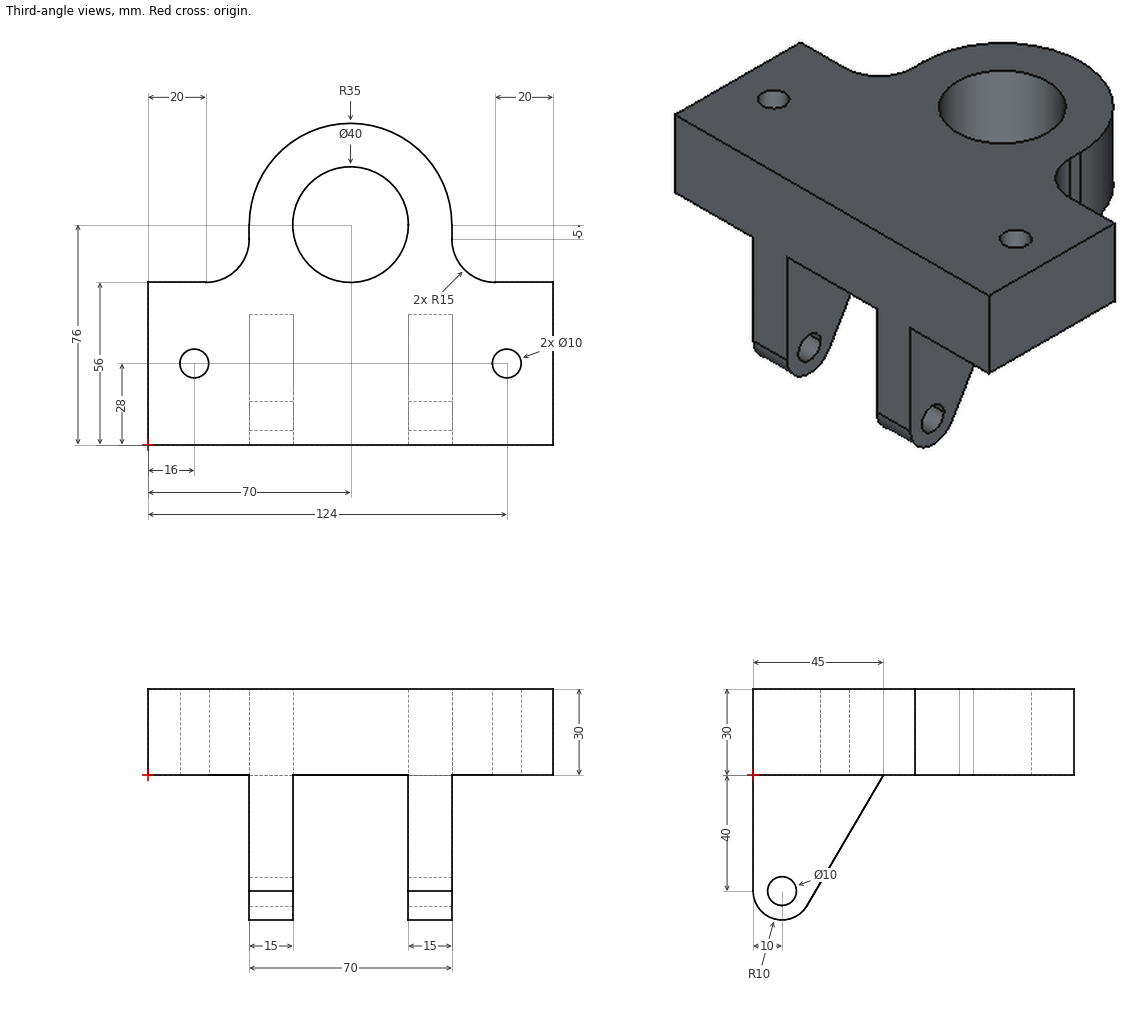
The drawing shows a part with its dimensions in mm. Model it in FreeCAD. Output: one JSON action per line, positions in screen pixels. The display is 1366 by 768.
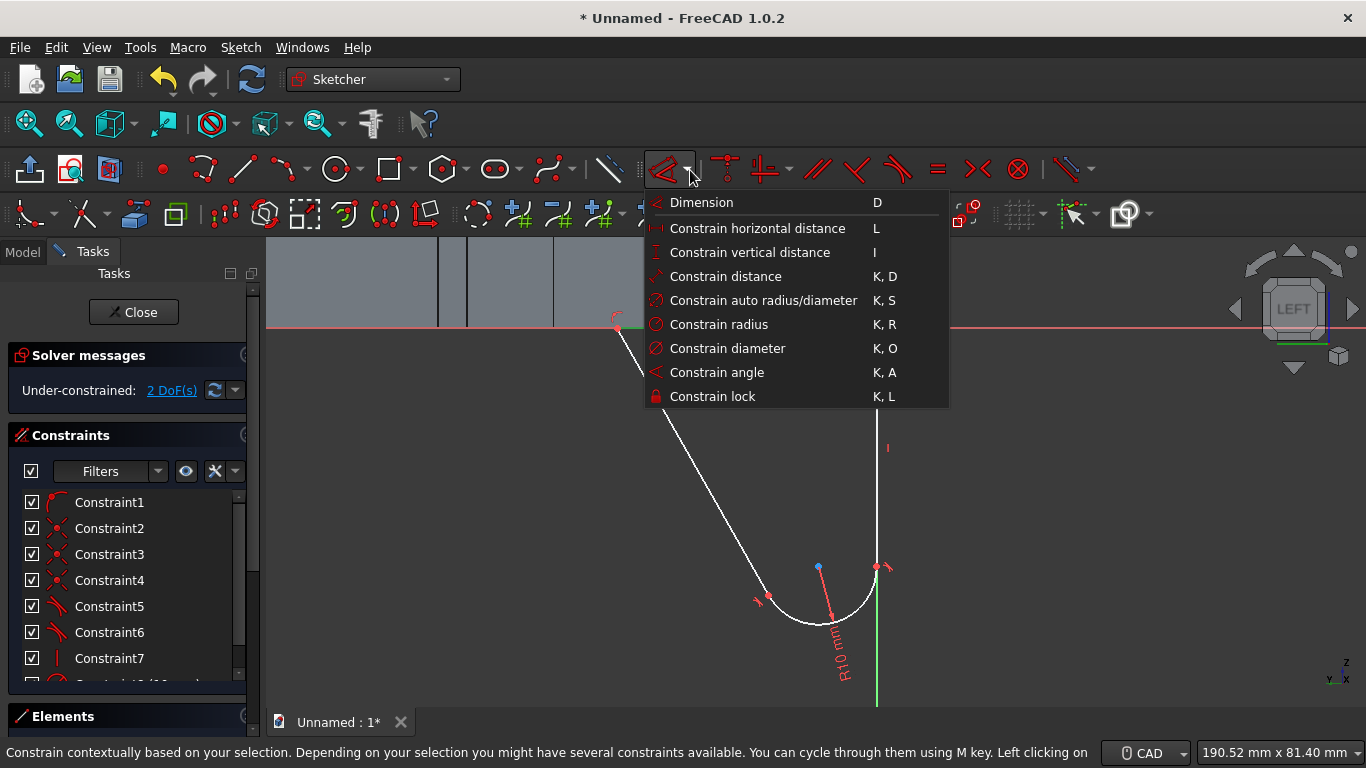
{"action": "left_click", "coordinate": [797, 228]}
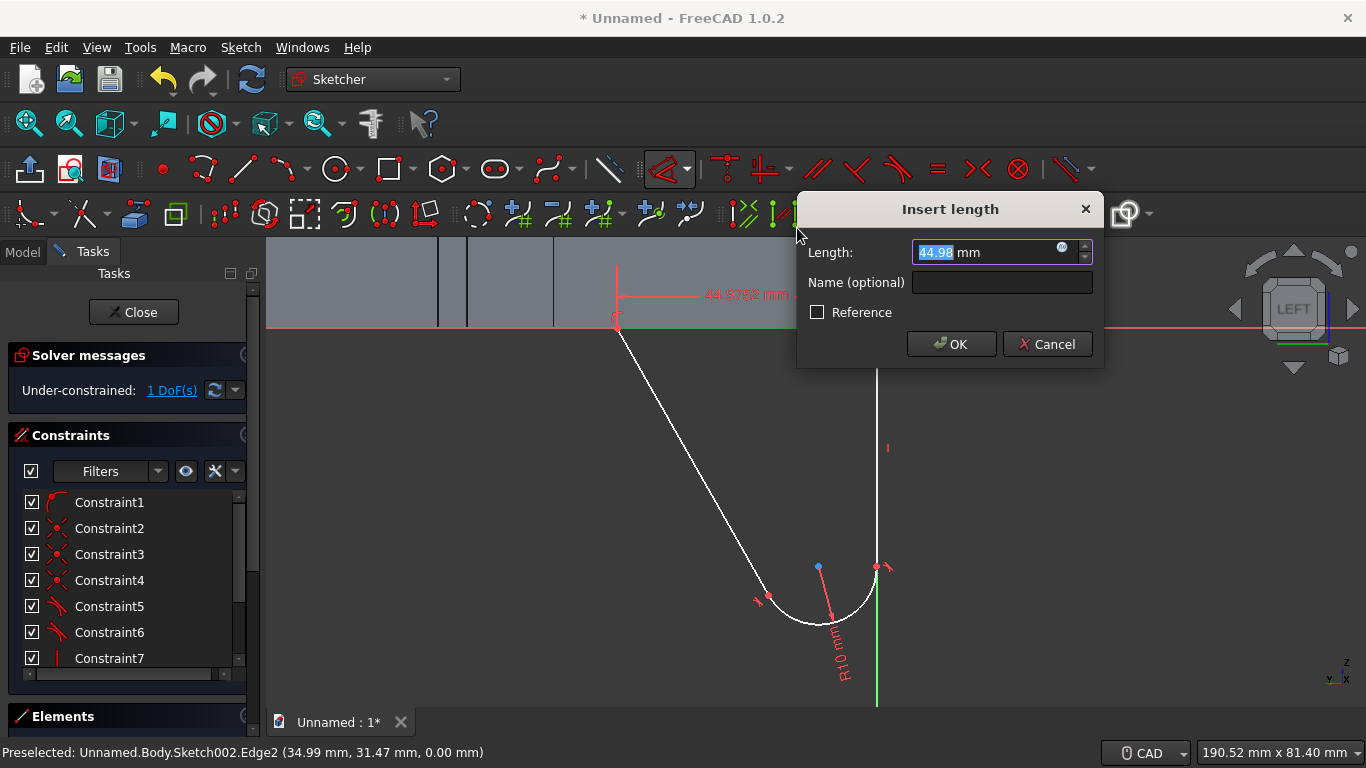
{"action": "type", "text": "45"}
{"action": "key", "text": "Return"}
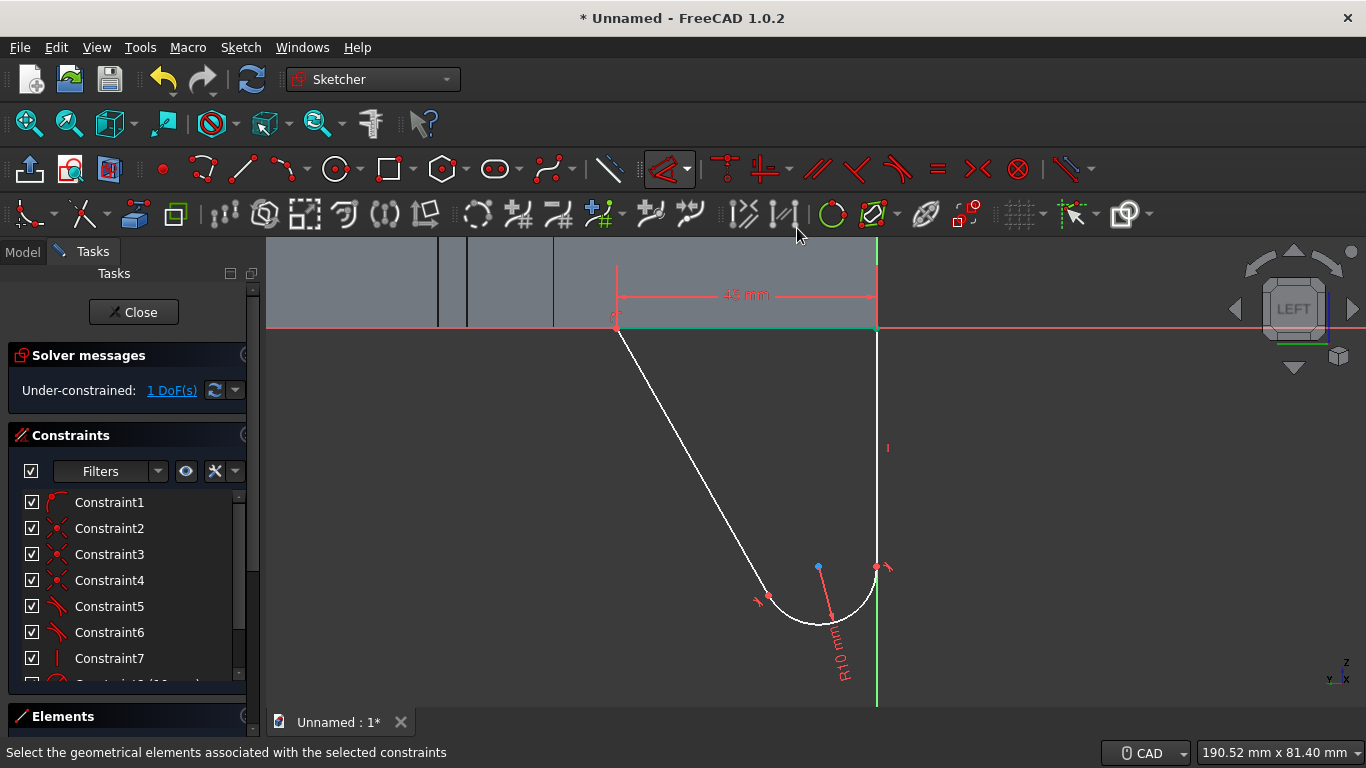
{"action": "left_click", "coordinate": [877, 400]}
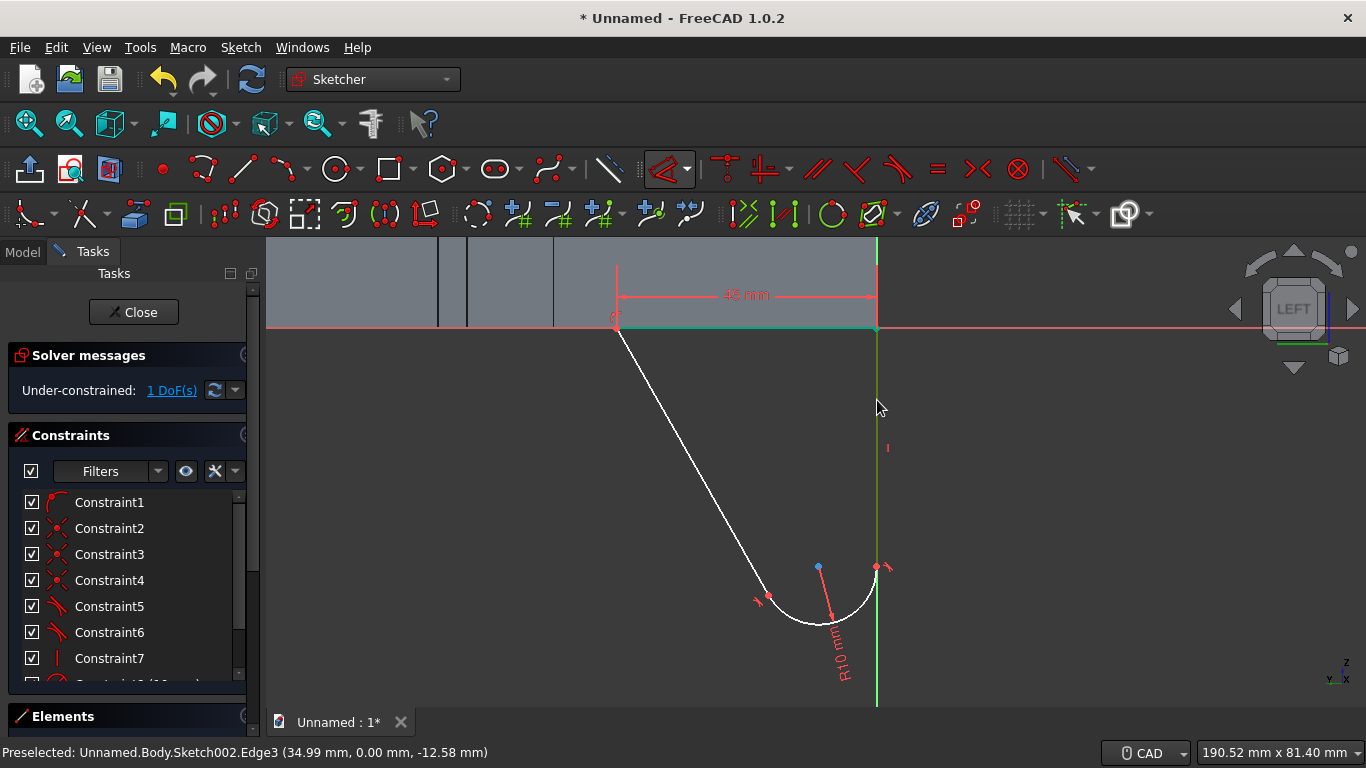
{"action": "left_click", "coordinate": [690, 170]}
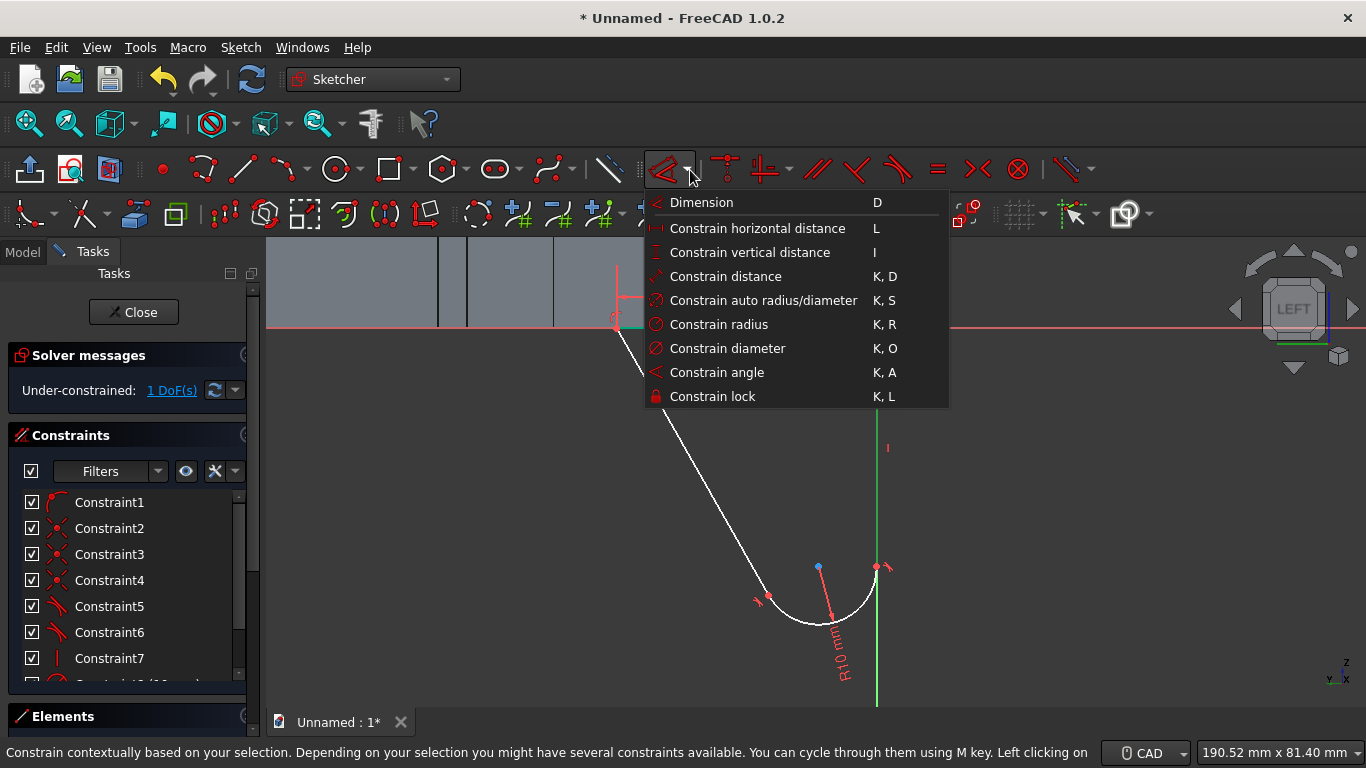
{"action": "left_click", "coordinate": [797, 252]}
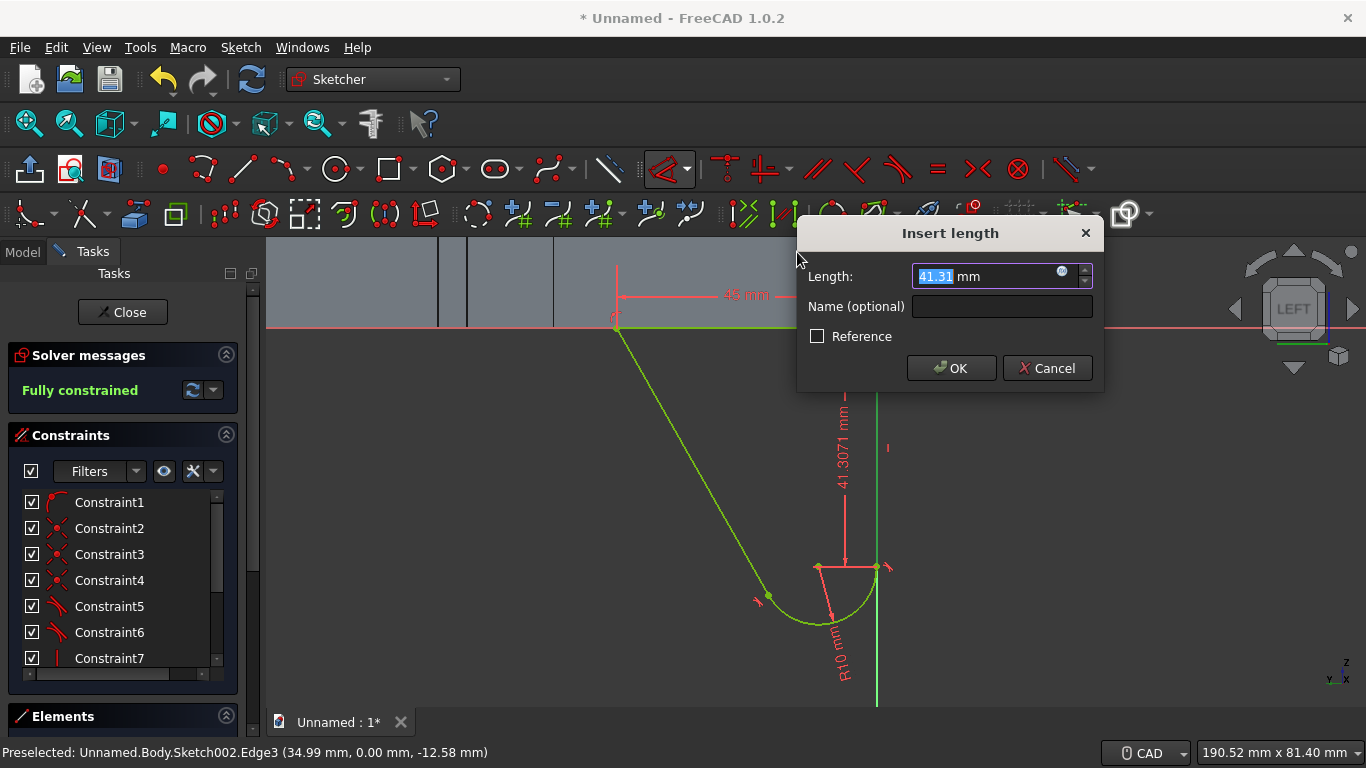
{"action": "type", "text": "40"}
{"action": "key", "text": "Return"}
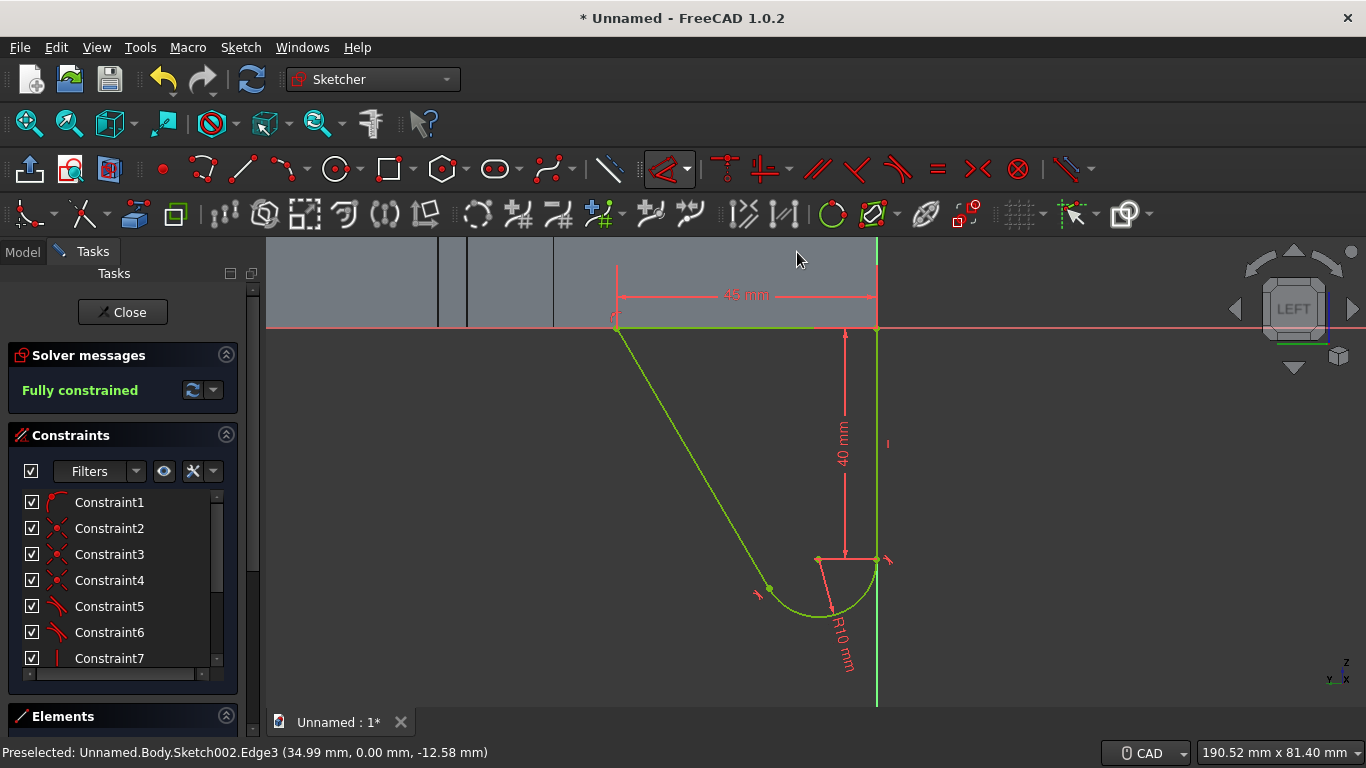
{"action": "left_click", "coordinate": [123, 312]}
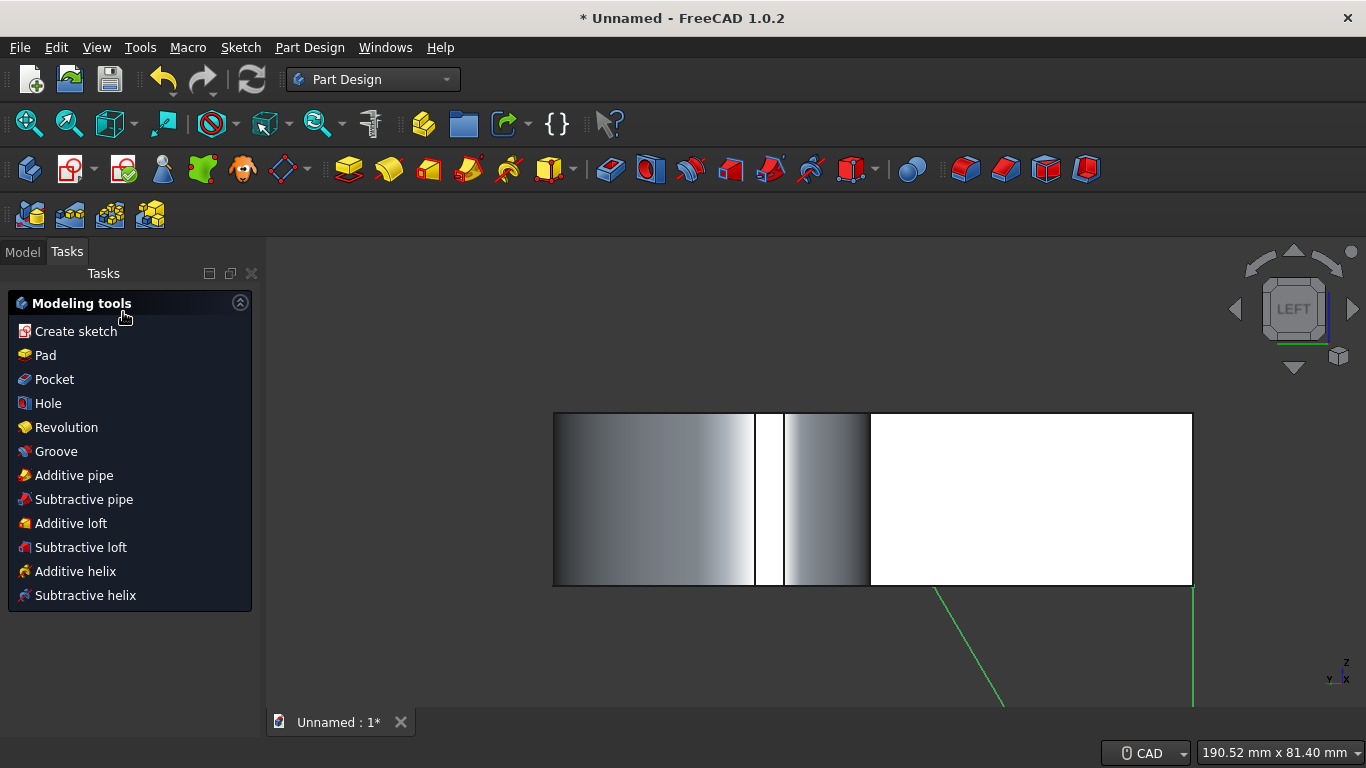
{"action": "left_click", "coordinate": [350, 170]}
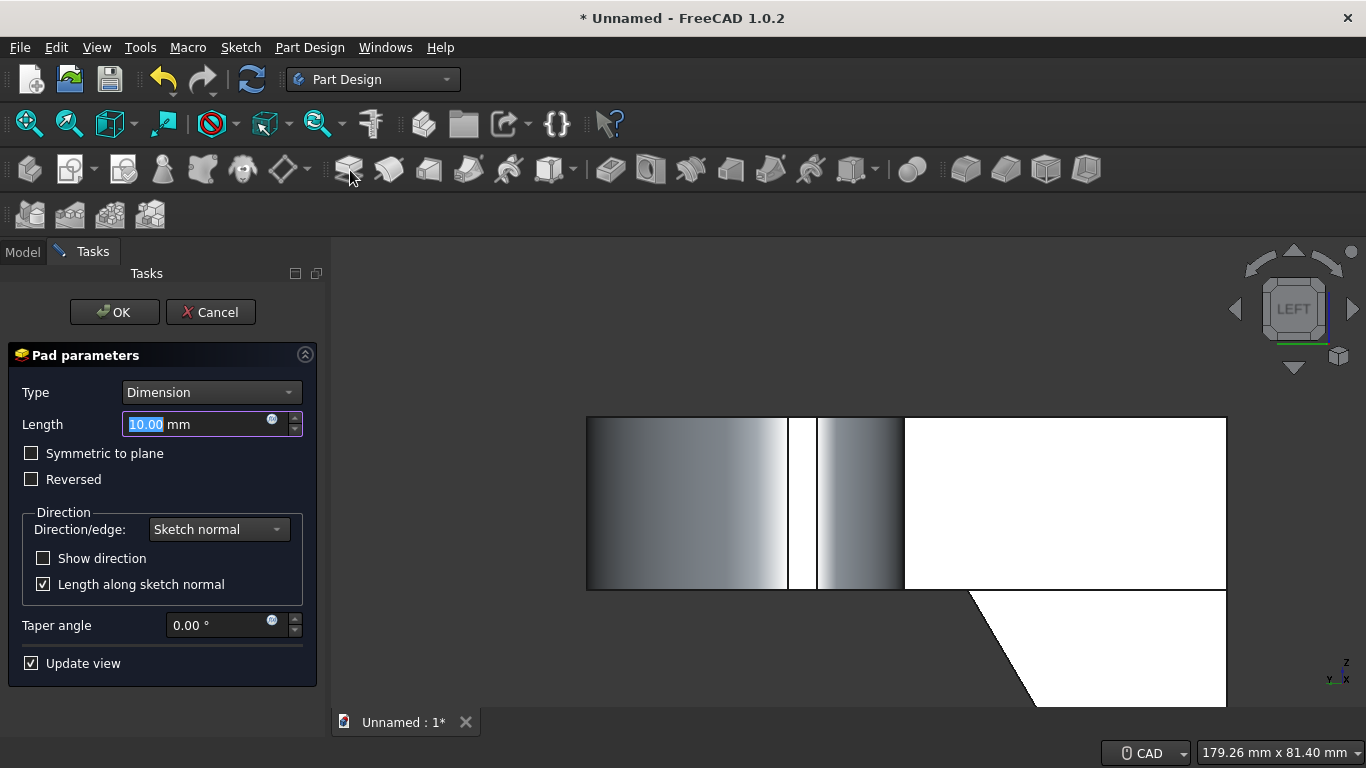
{"action": "type", "text": "15"}
{"action": "key", "text": "Tab"}